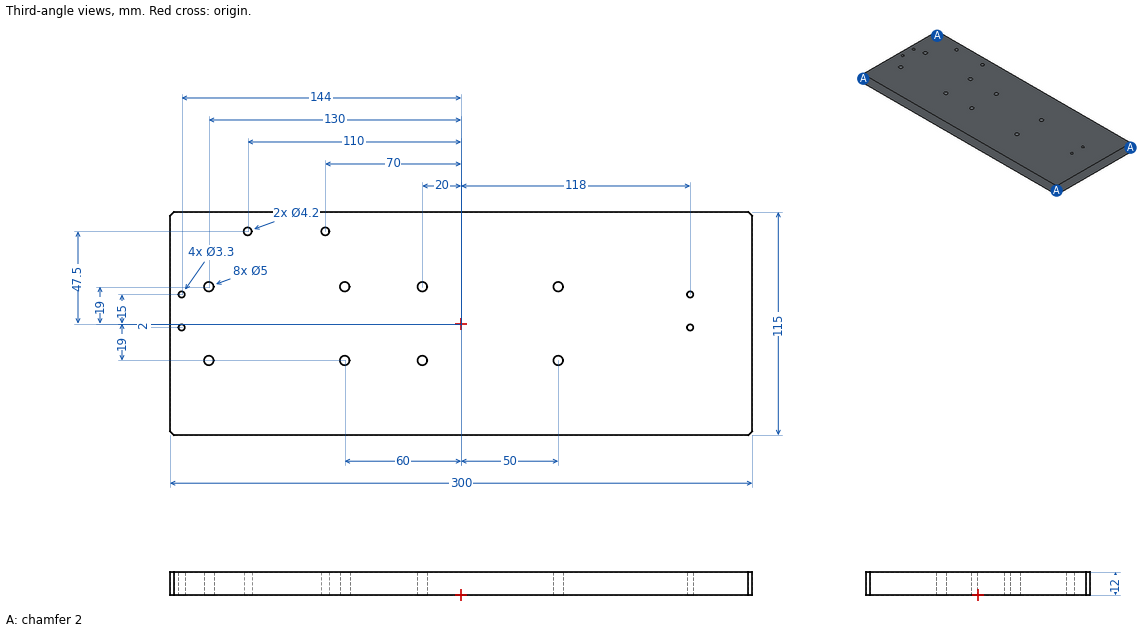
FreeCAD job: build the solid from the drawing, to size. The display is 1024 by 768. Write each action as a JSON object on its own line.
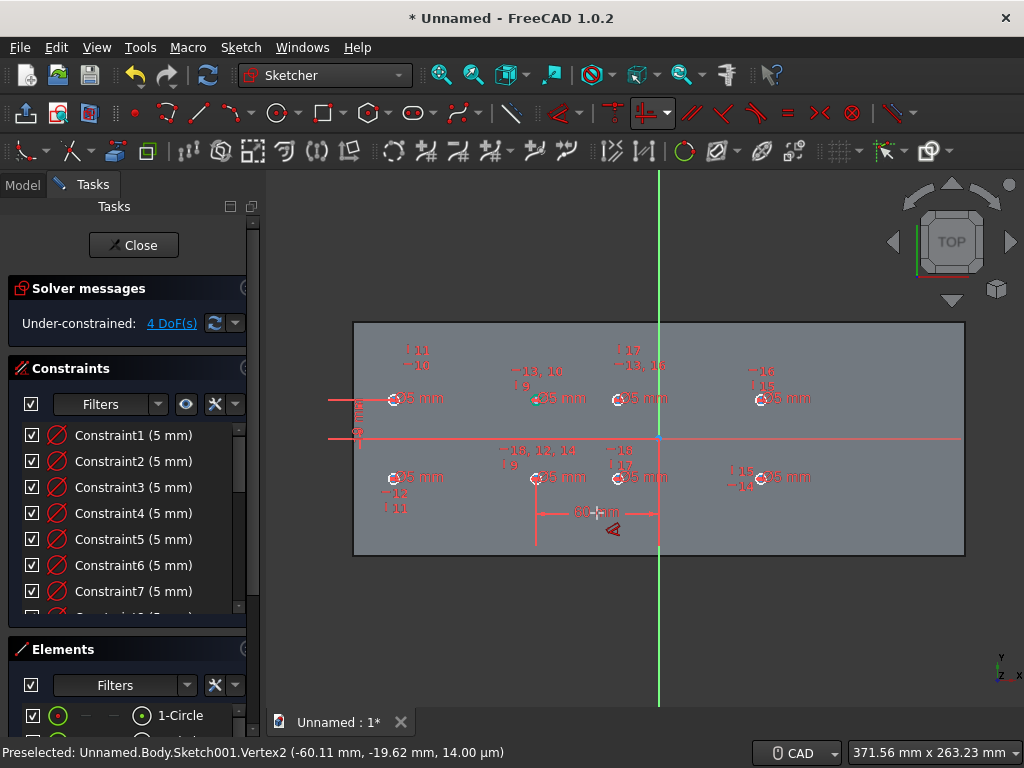
{"action": "left_click", "coordinate": [536, 479]}
{"action": "left_click", "coordinate": [693, 459]}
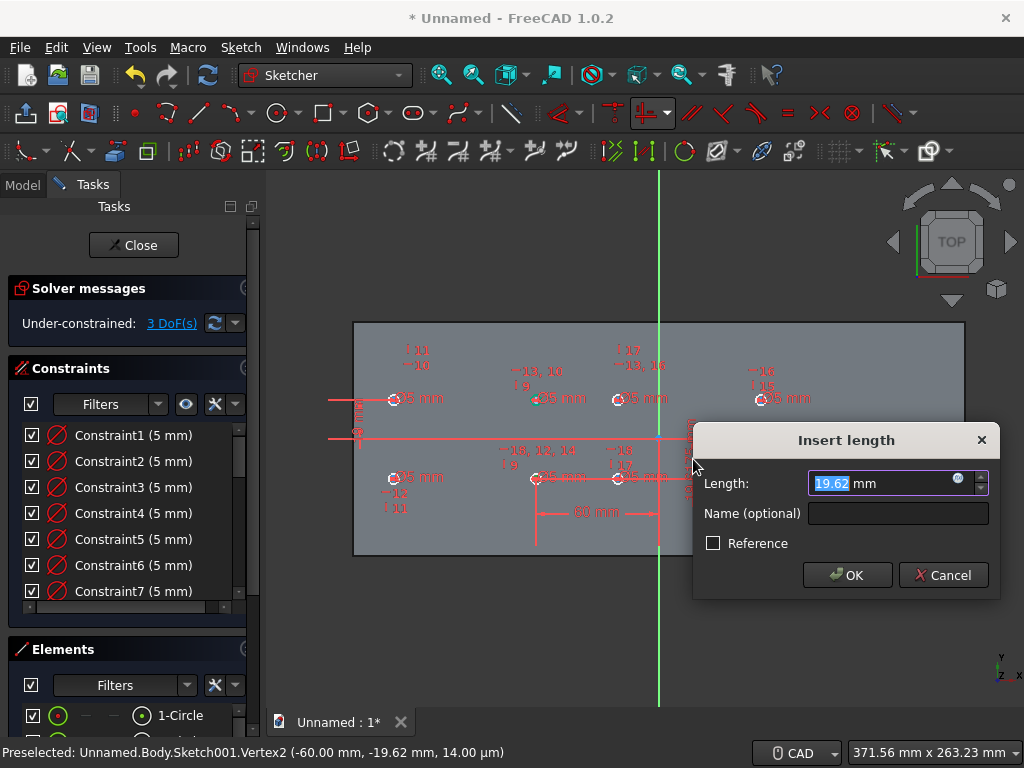
{"action": "type", "text": "19"}
{"action": "key", "text": "Return"}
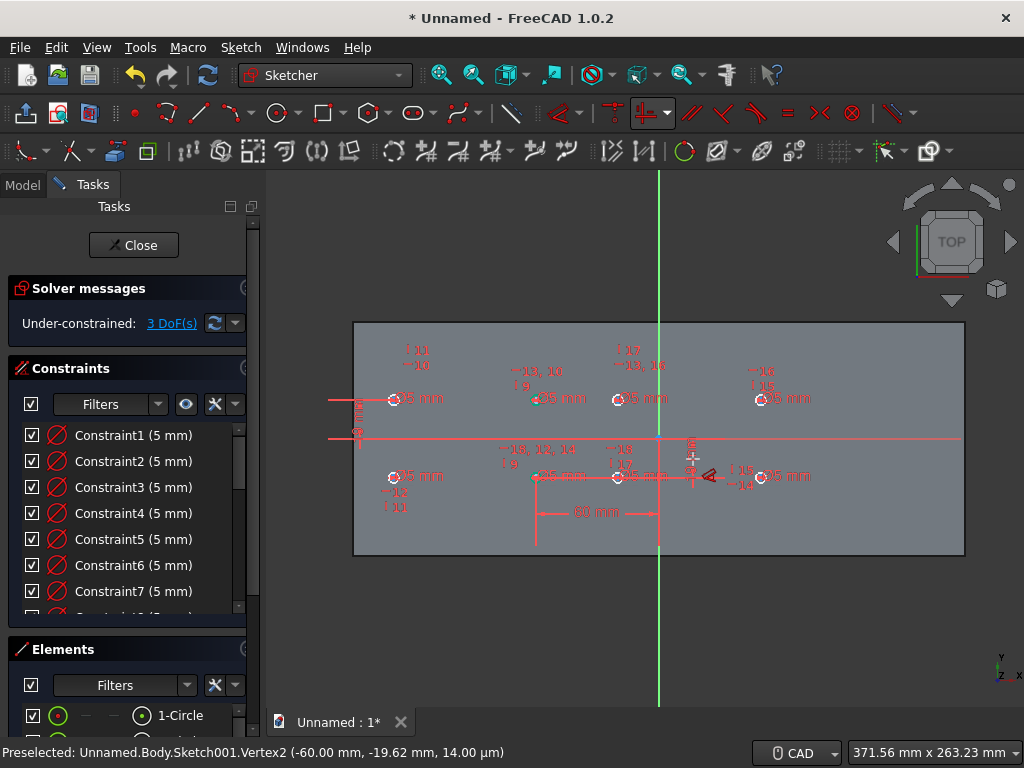
{"action": "left_click", "coordinate": [618, 400]}
{"action": "left_click", "coordinate": [638, 366]}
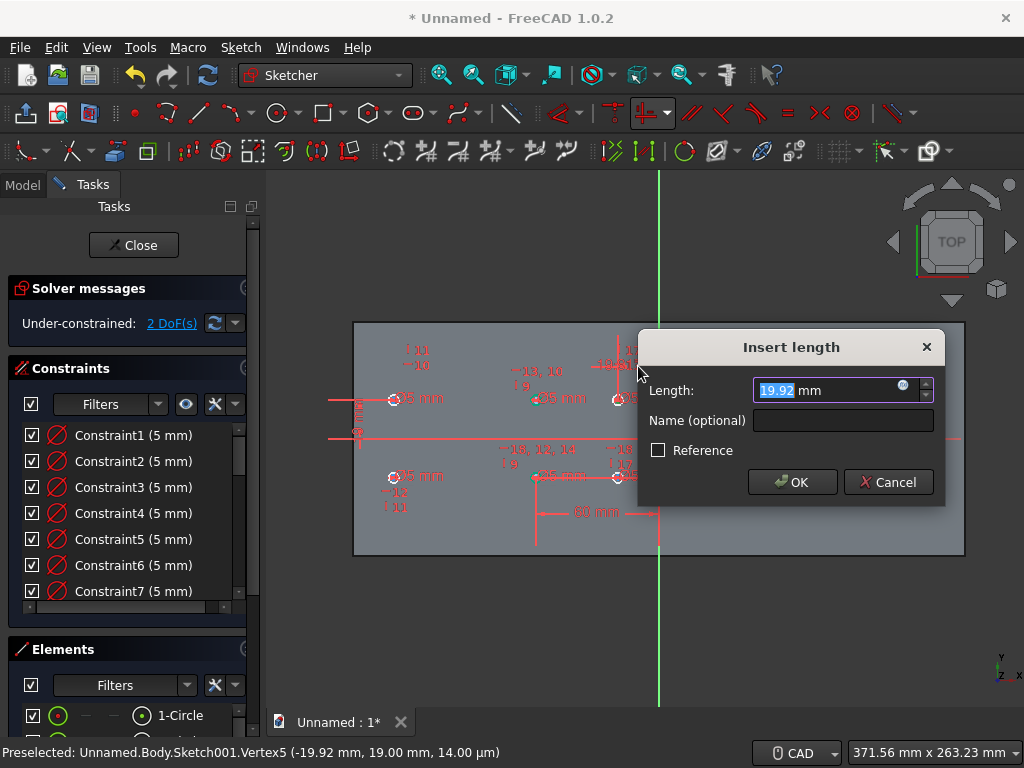
{"action": "type", "text": "20"}
{"action": "key", "text": "Return"}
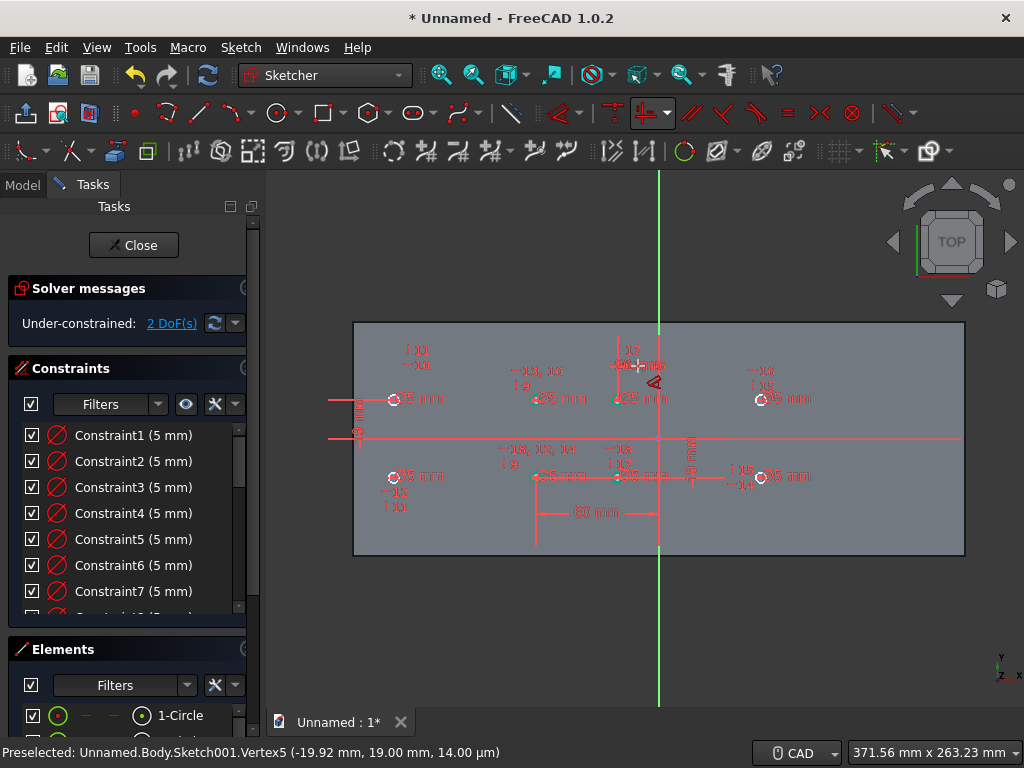
{"action": "left_click", "coordinate": [761, 478]}
{"action": "left_click", "coordinate": [710, 512]}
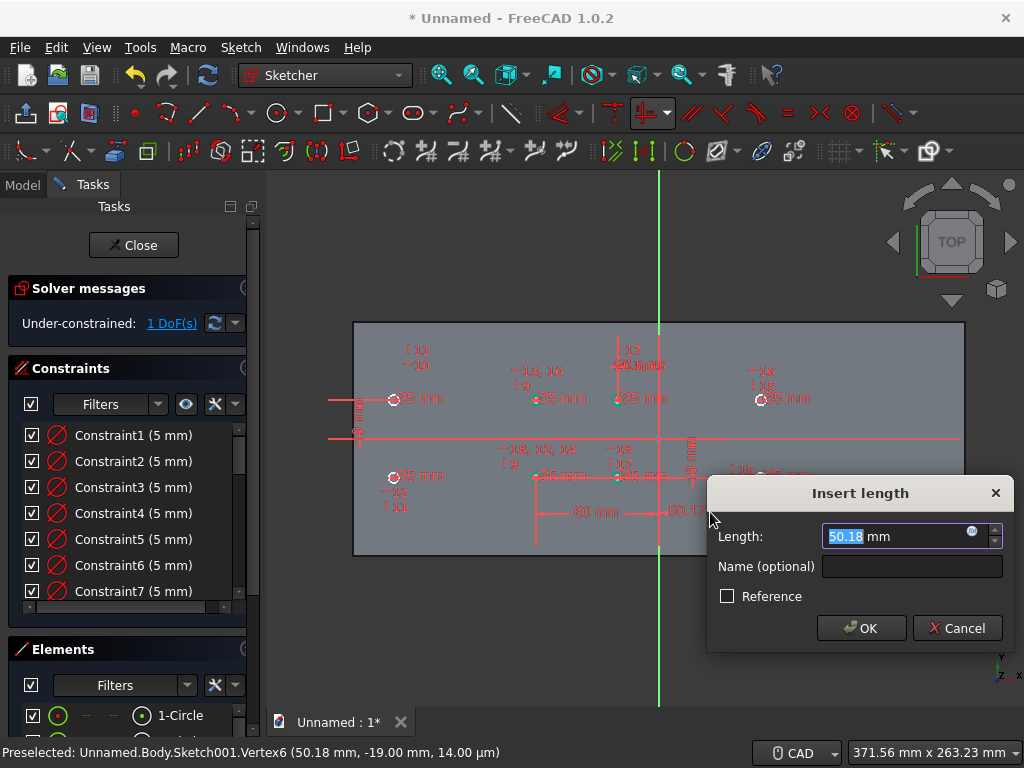
{"action": "type", "text": "50"}
{"action": "key", "text": "Return"}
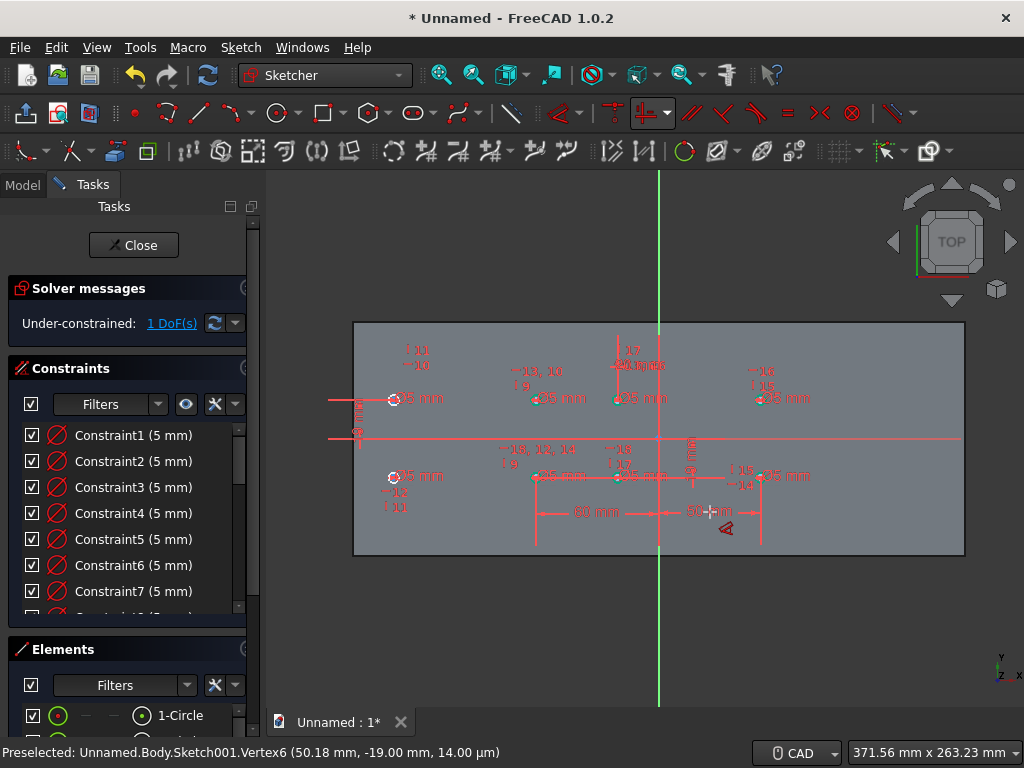
{"action": "left_click", "coordinate": [394, 400]}
{"action": "left_click", "coordinate": [526, 366]}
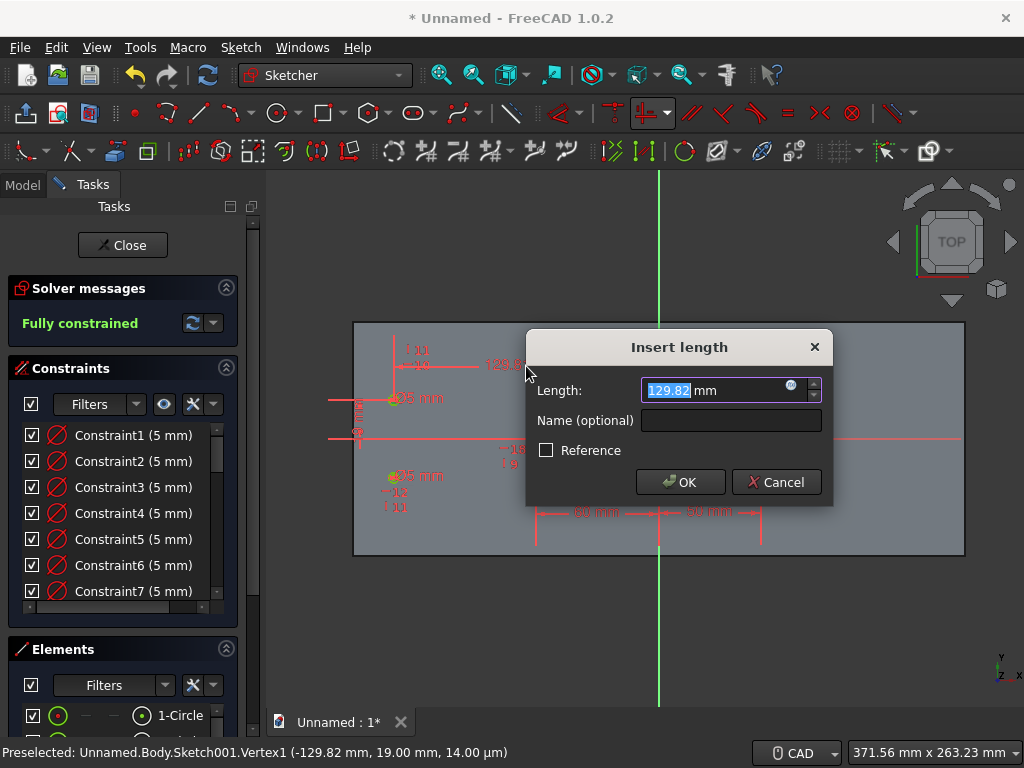
{"action": "type", "text": "130"}
{"action": "key", "text": "Return"}
{"action": "key", "text": "Escape"}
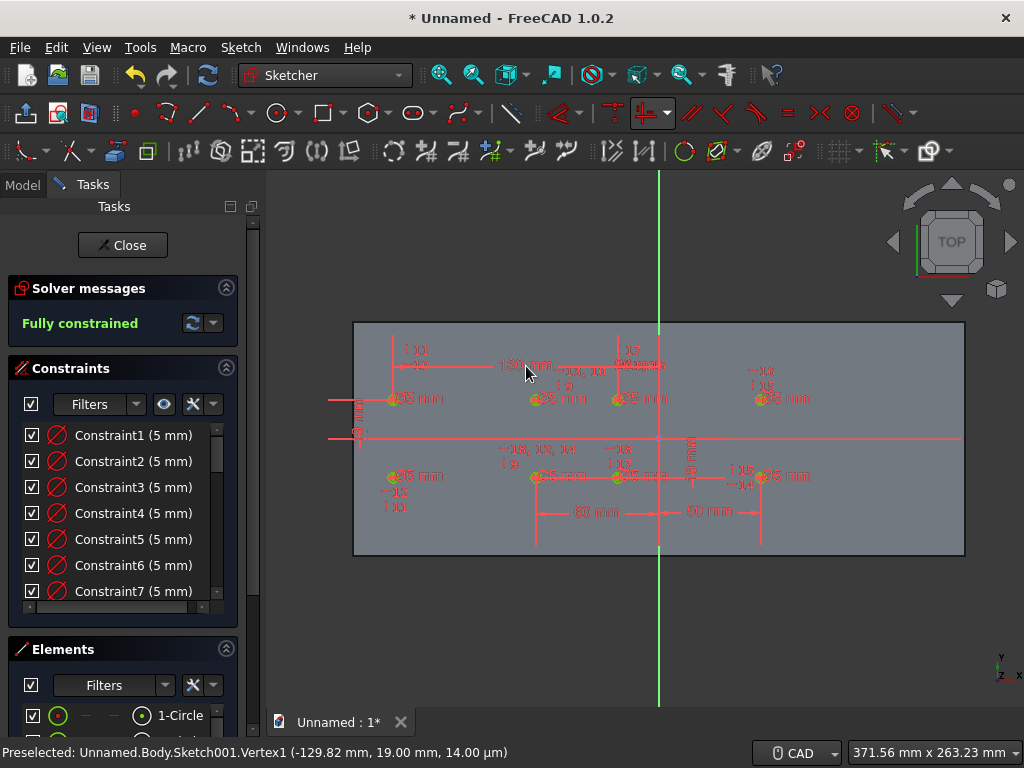
{"action": "left_click", "coordinate": [123, 245]}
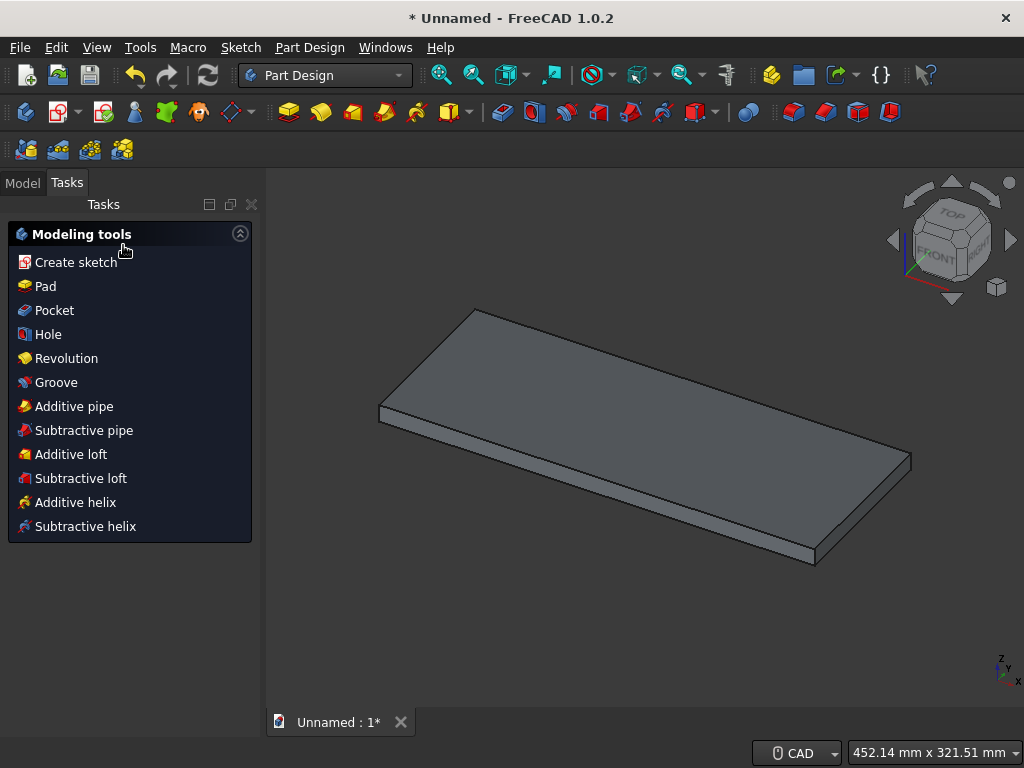
{"action": "left_click", "coordinate": [504, 112]}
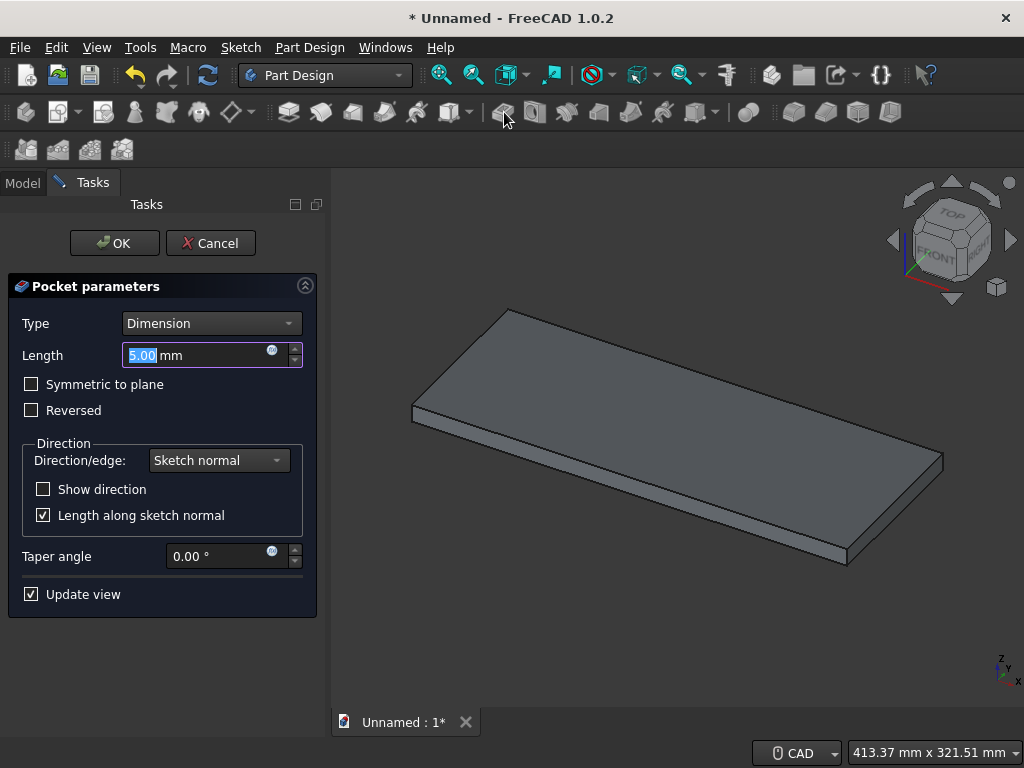
{"action": "left_click", "coordinate": [212, 324]}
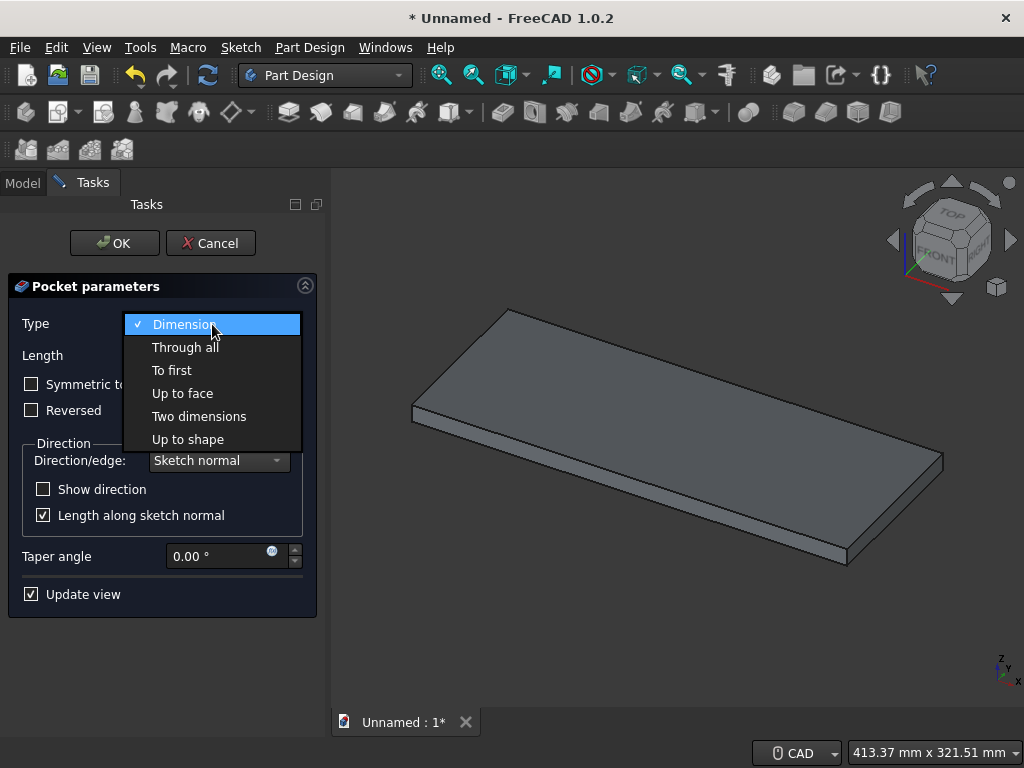
{"action": "left_click", "coordinate": [212, 348]}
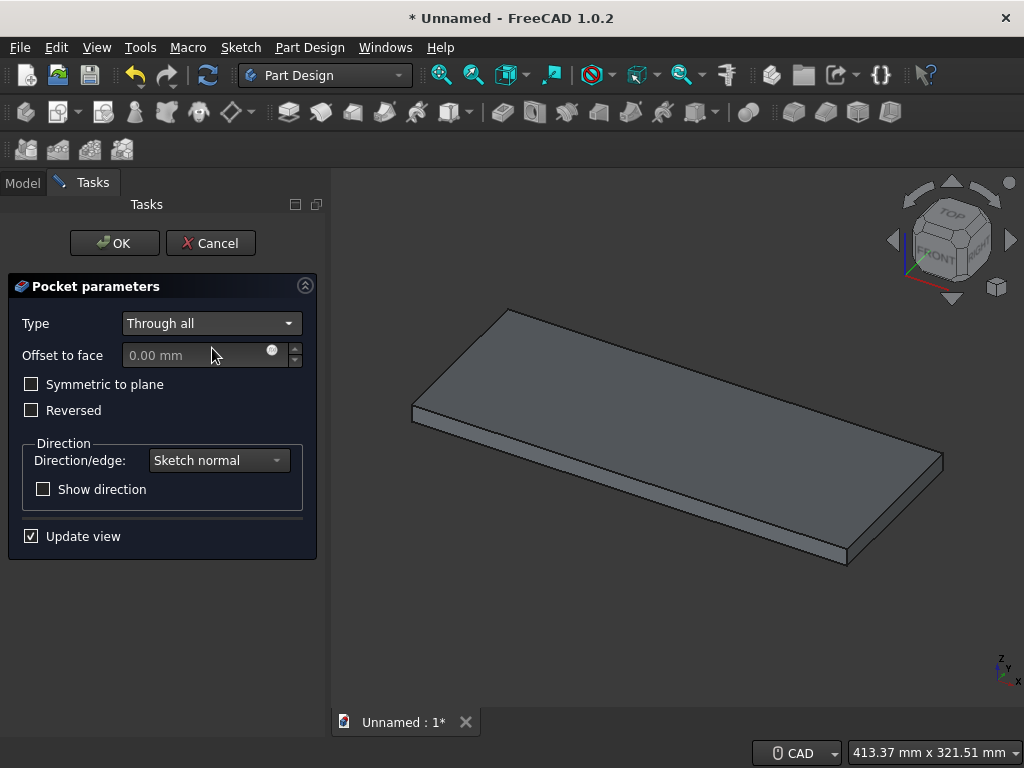
{"action": "left_click", "coordinate": [30, 410]}